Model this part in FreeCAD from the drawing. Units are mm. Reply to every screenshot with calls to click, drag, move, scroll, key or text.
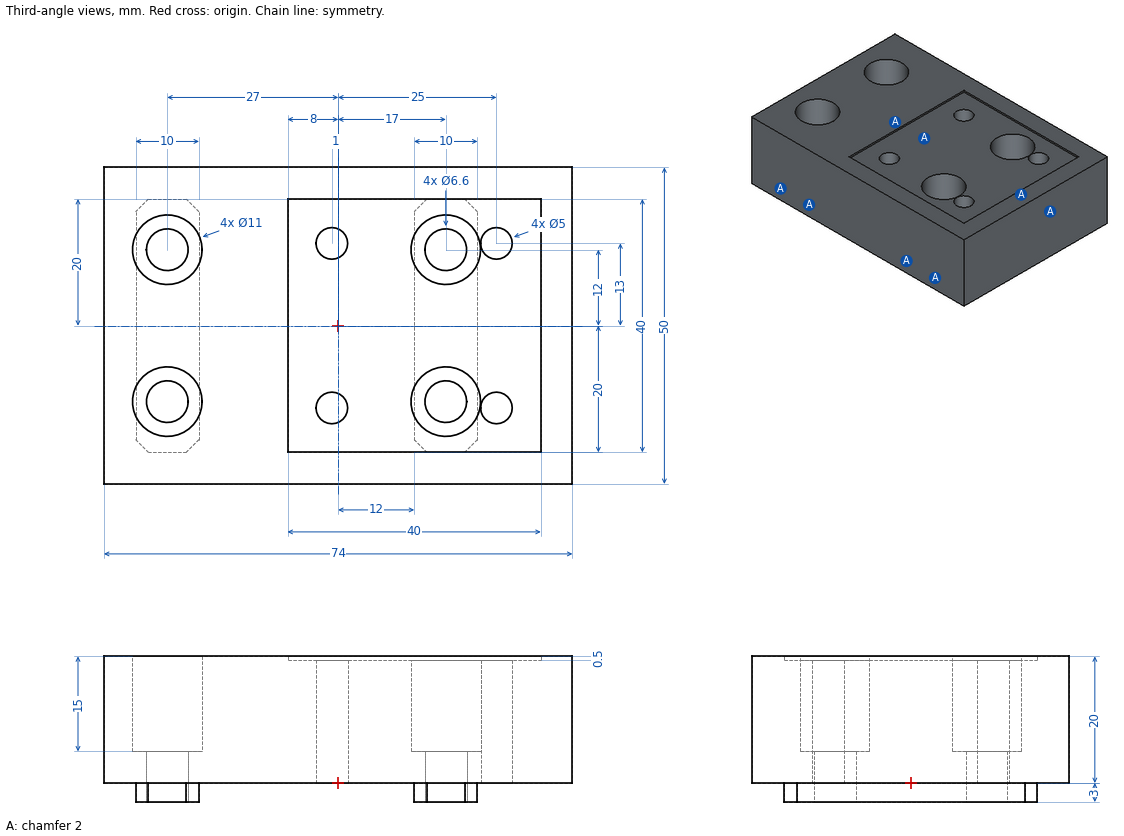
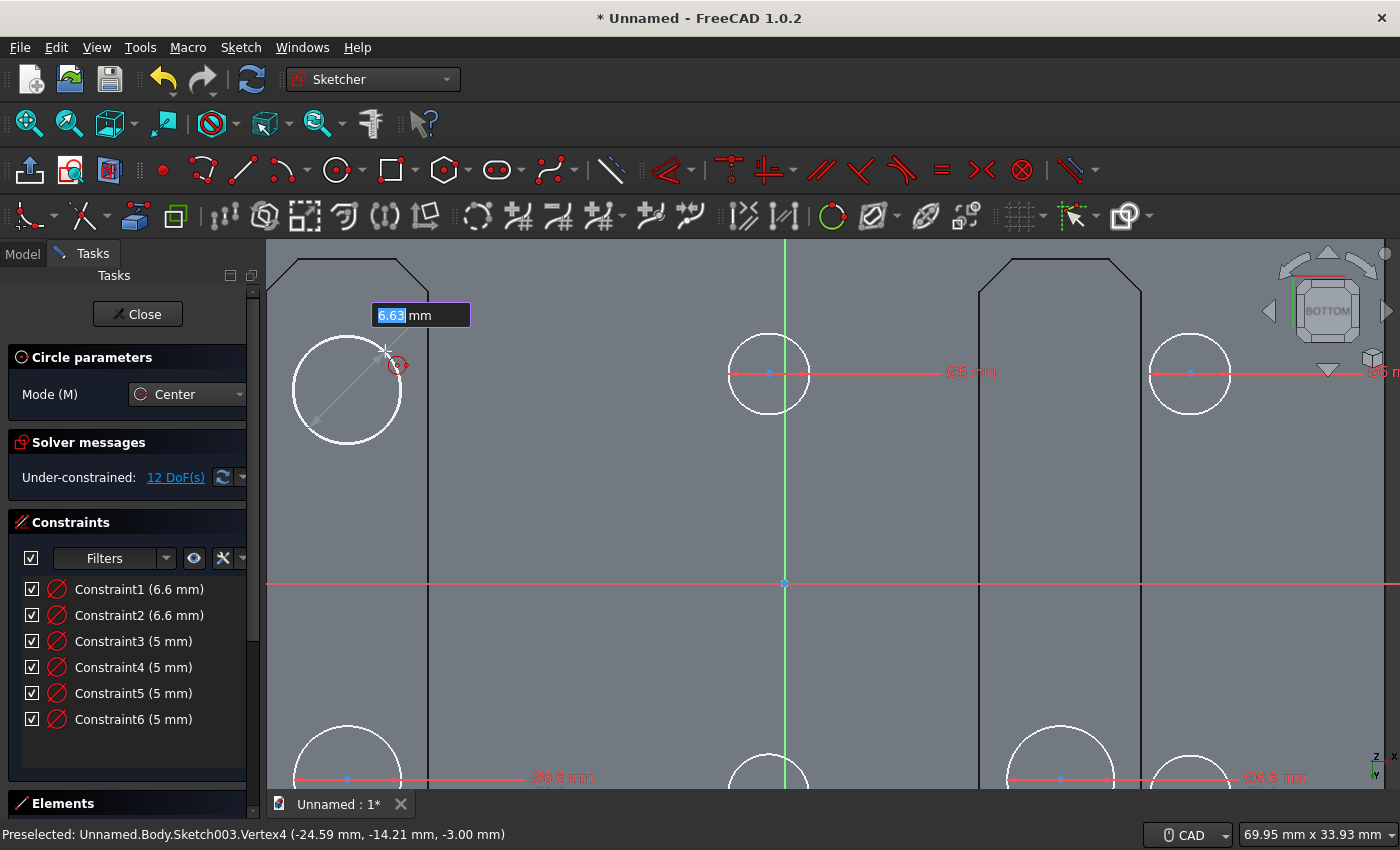
text(6.6)
key(Return)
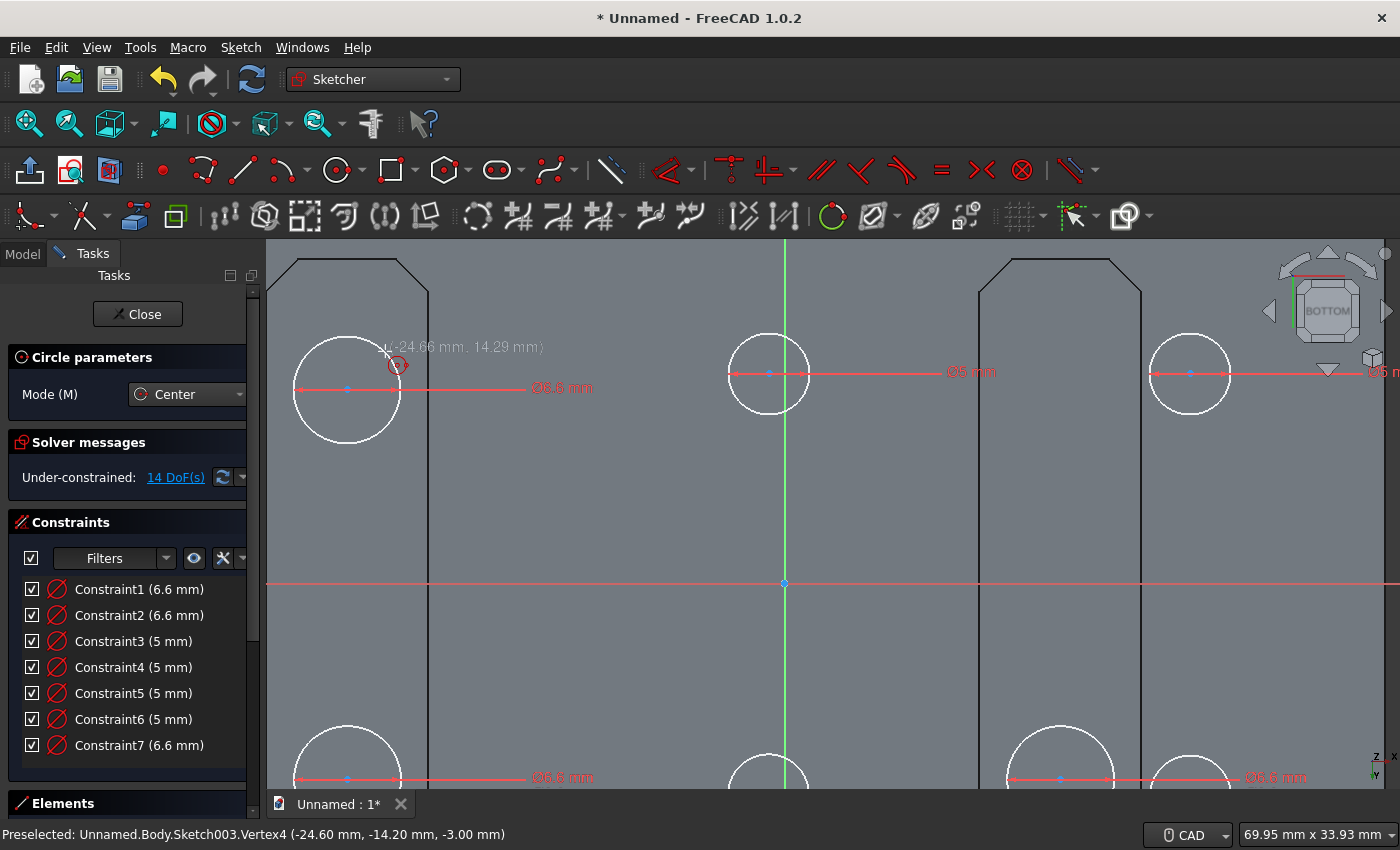
click(1060, 389)
move(1098, 351)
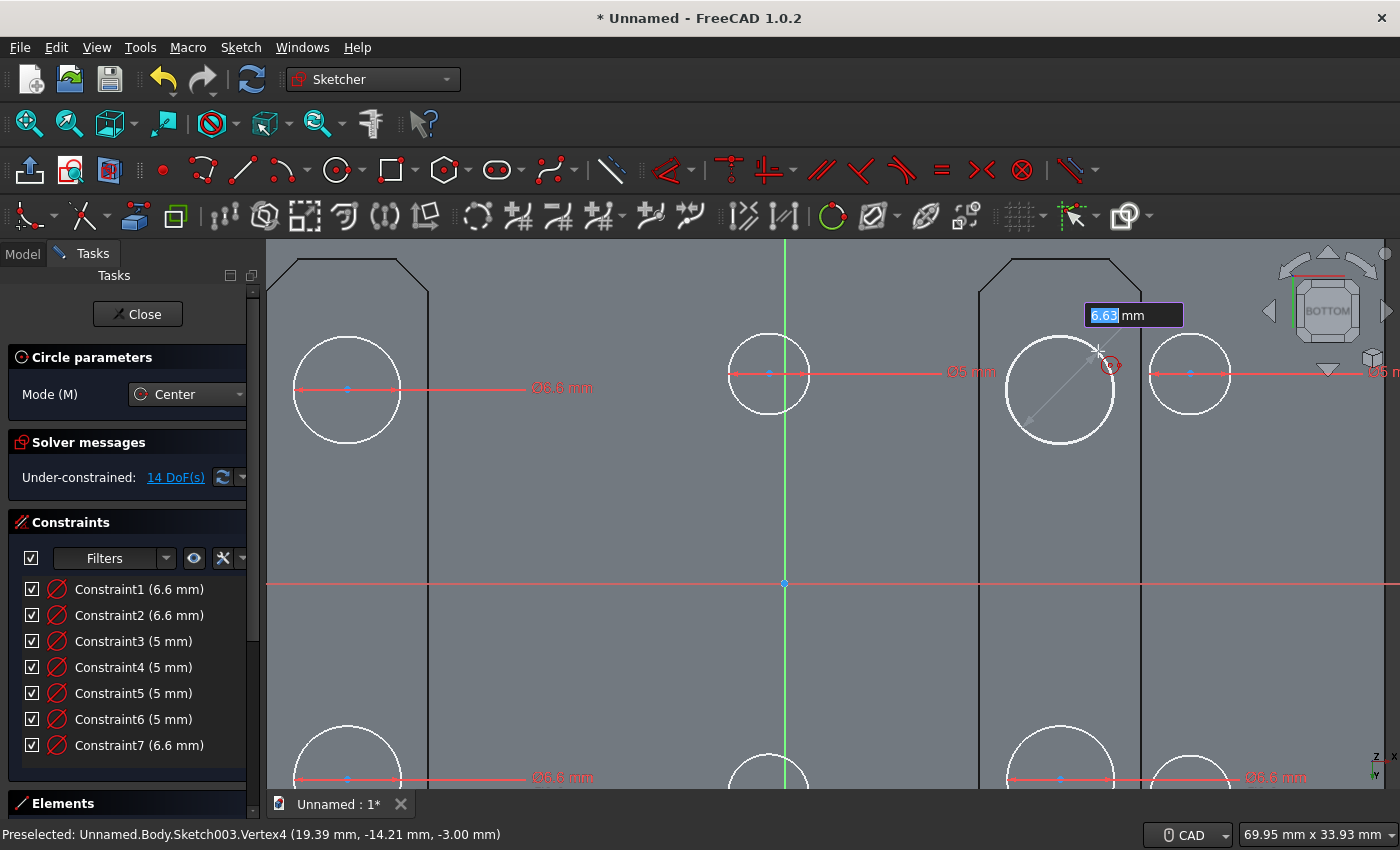
text(6.6)
key(Return)
key(Escape)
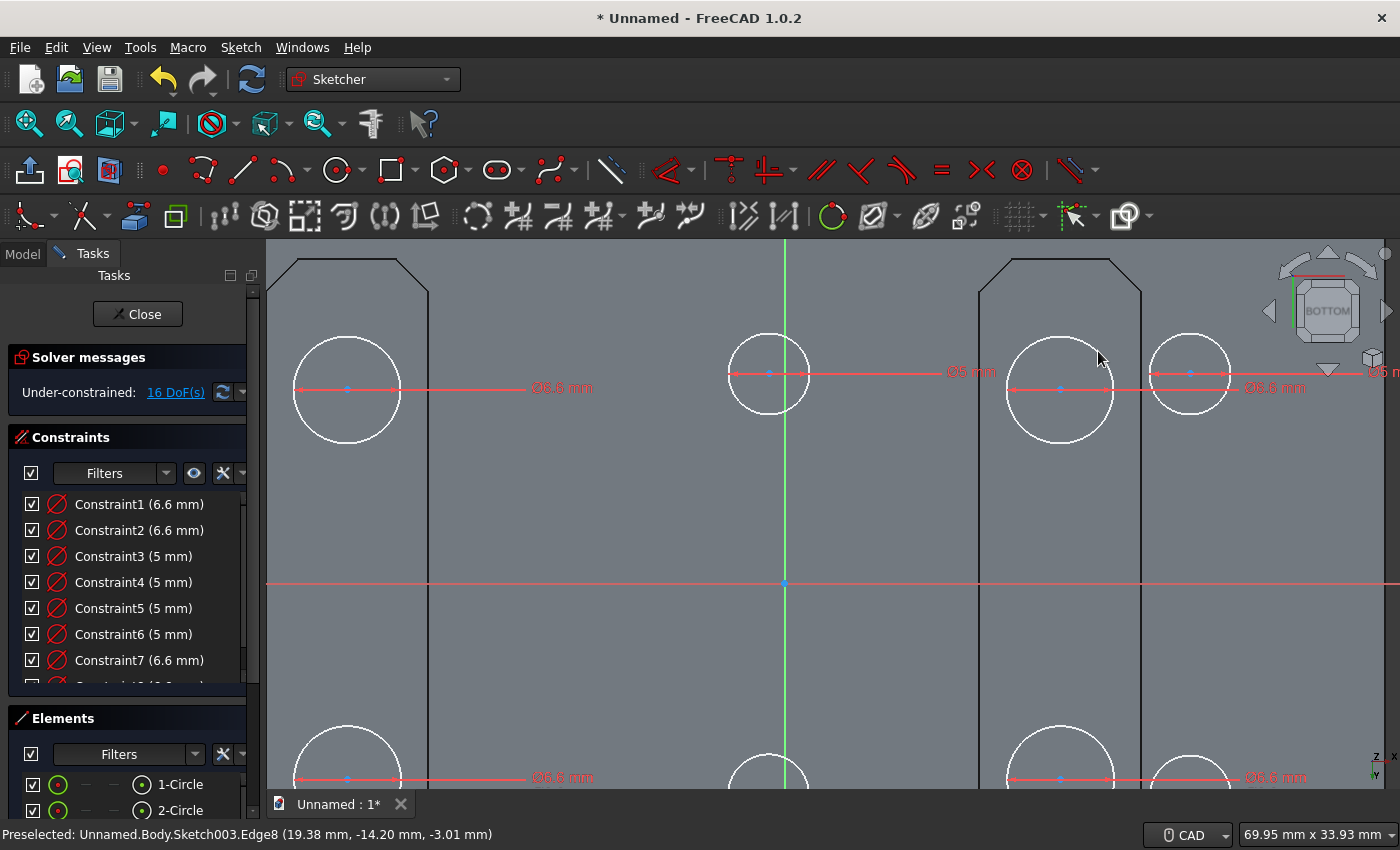
scroll(769, 372, down, 2)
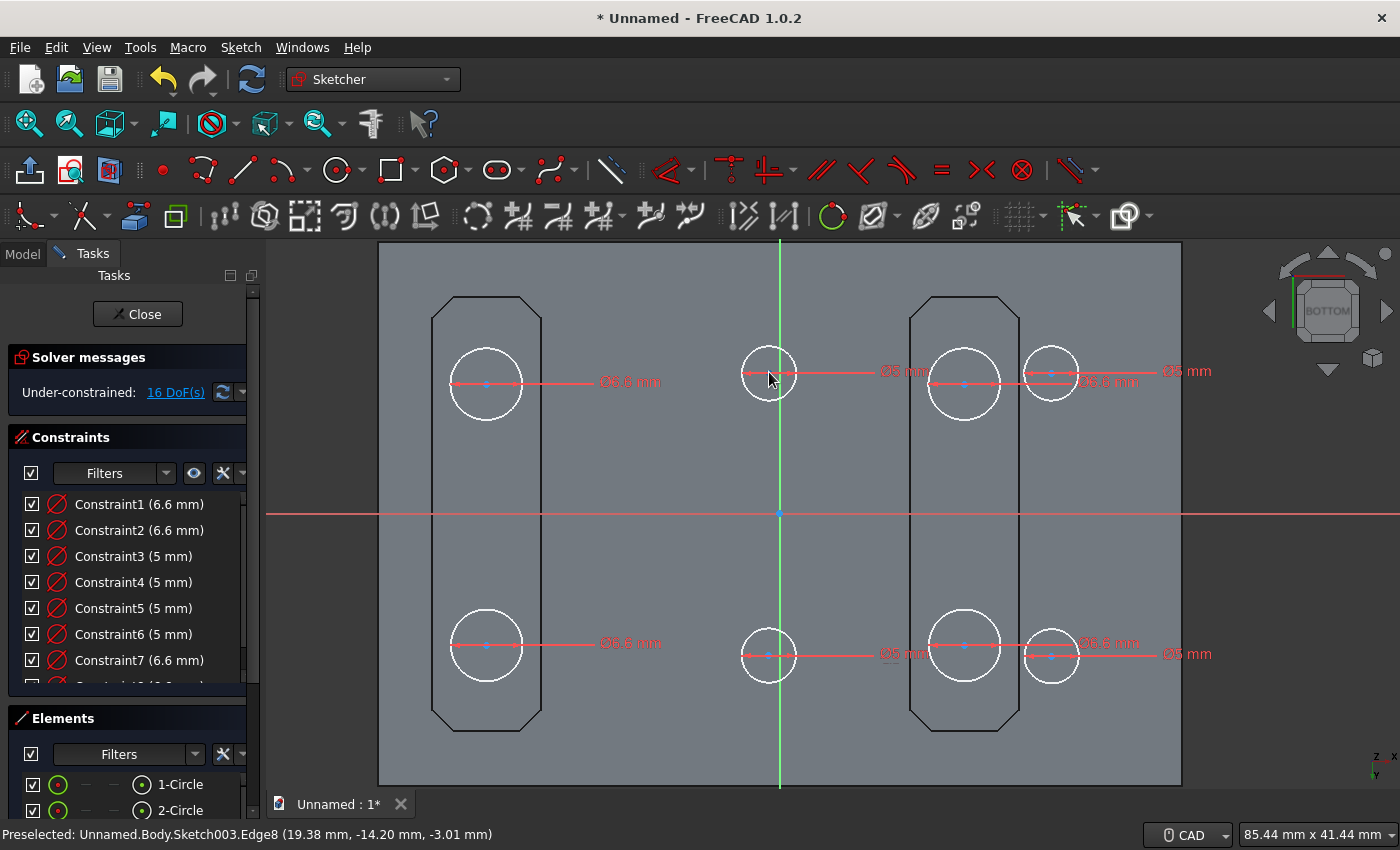
click(769, 656)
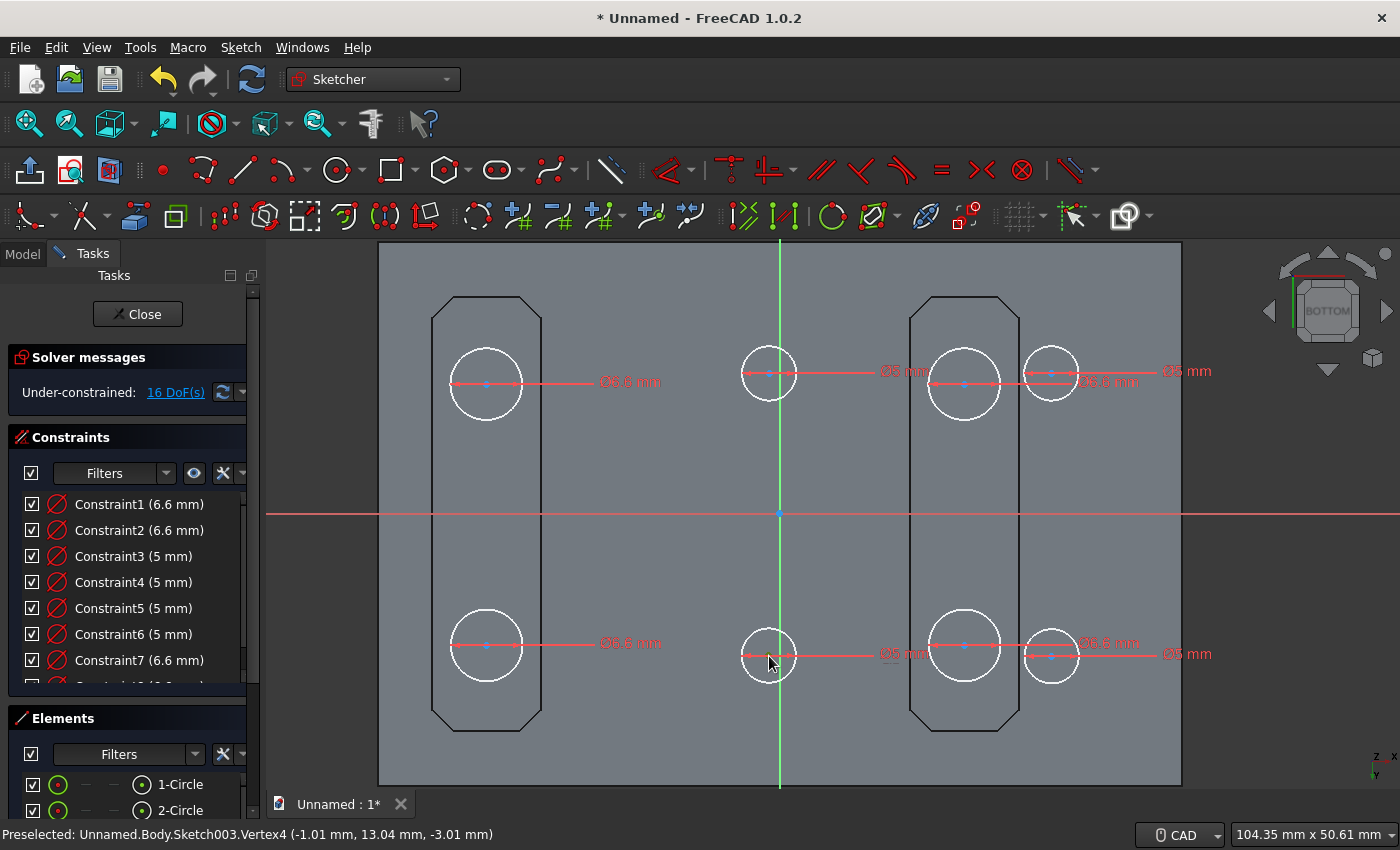
click(769, 373)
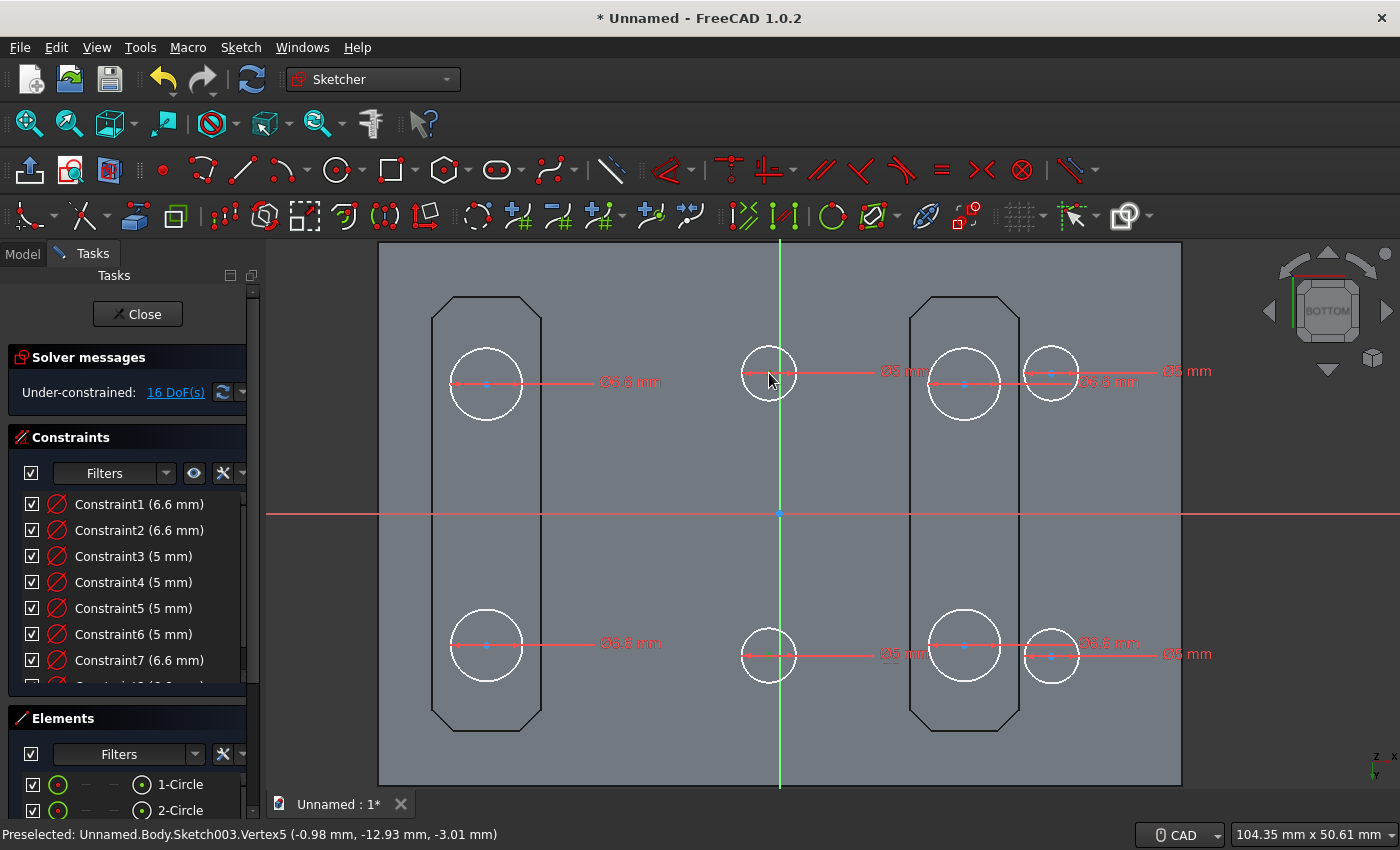
click(361, 514)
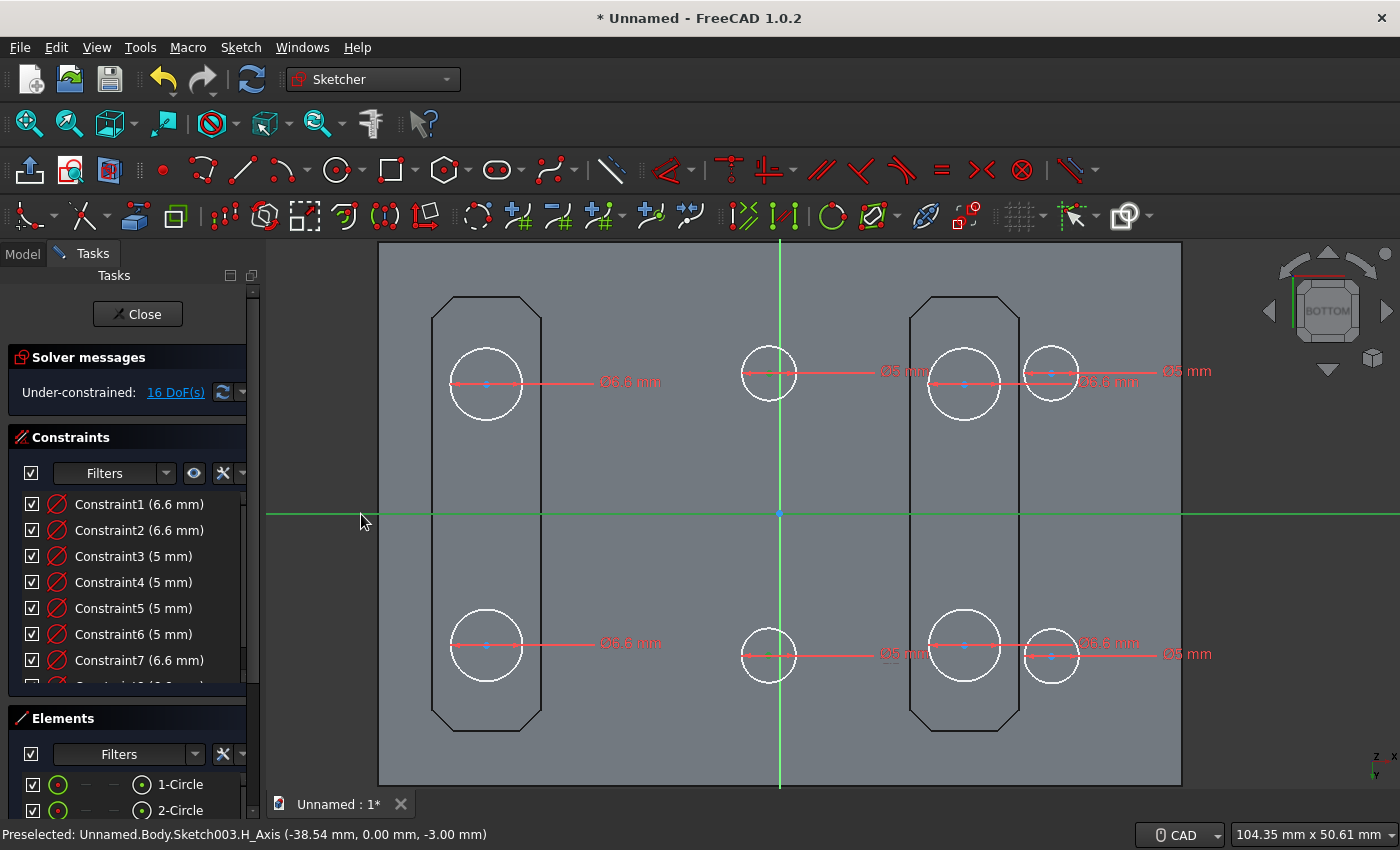
click(982, 170)